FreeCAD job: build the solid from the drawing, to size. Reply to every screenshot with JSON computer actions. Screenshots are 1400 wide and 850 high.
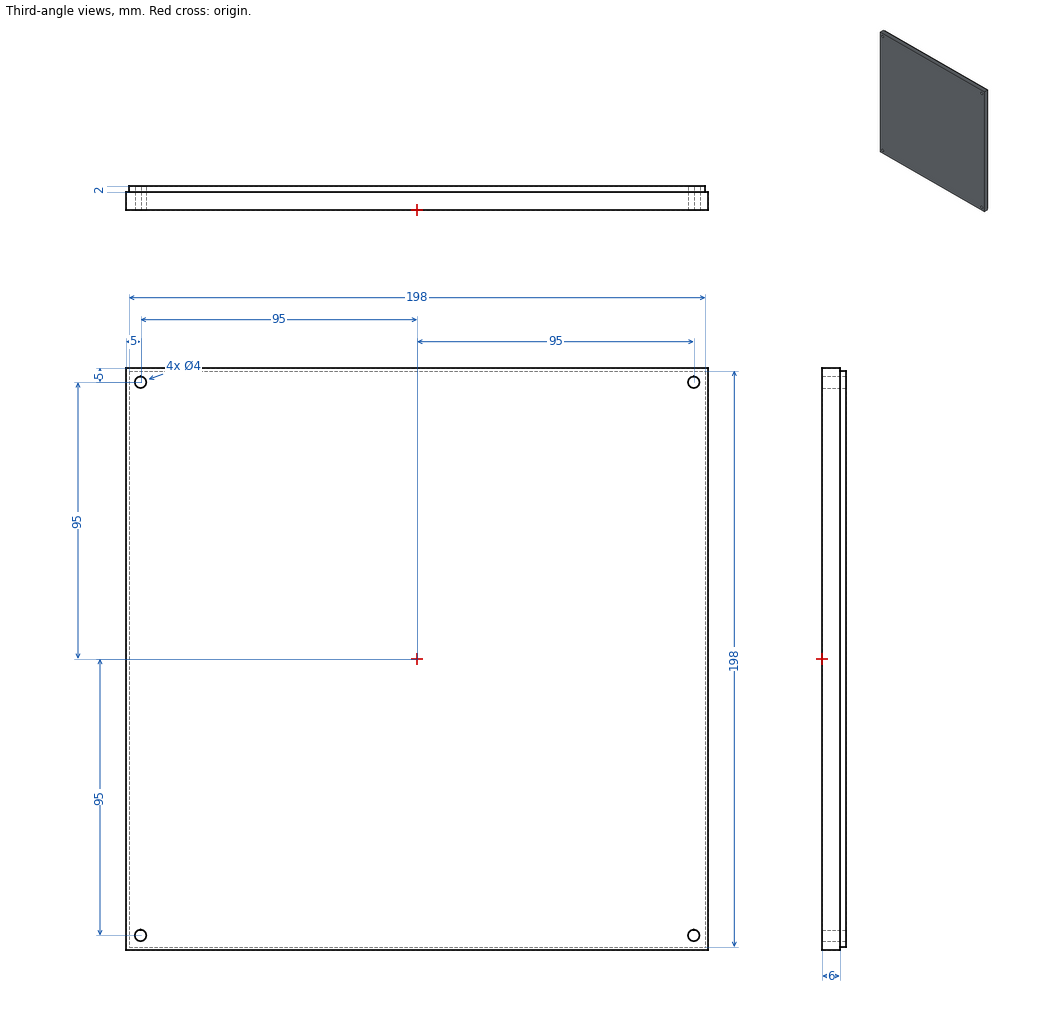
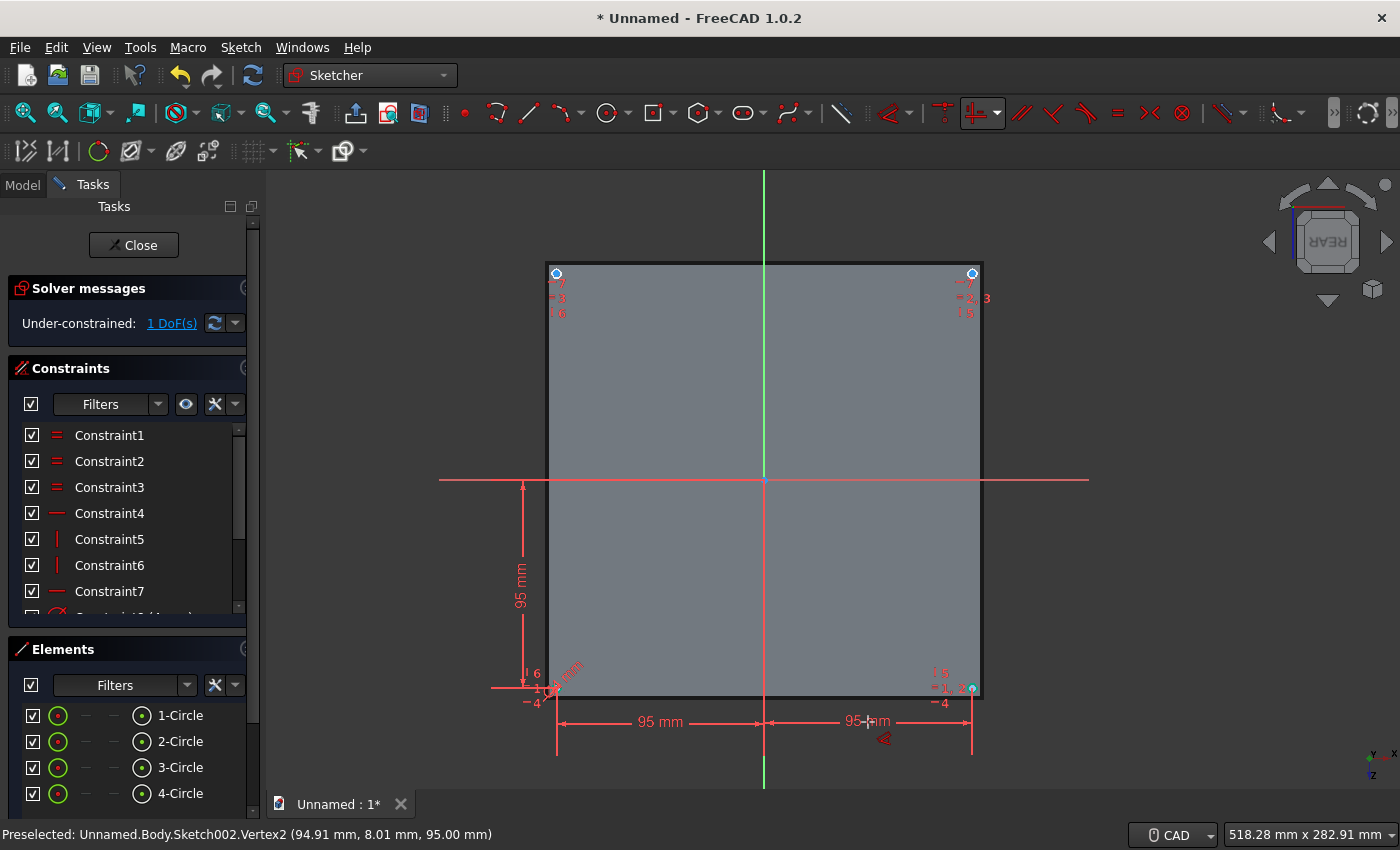
{"action": "left_click", "coordinate": [972, 274]}
{"action": "left_click", "coordinate": [1006, 377]}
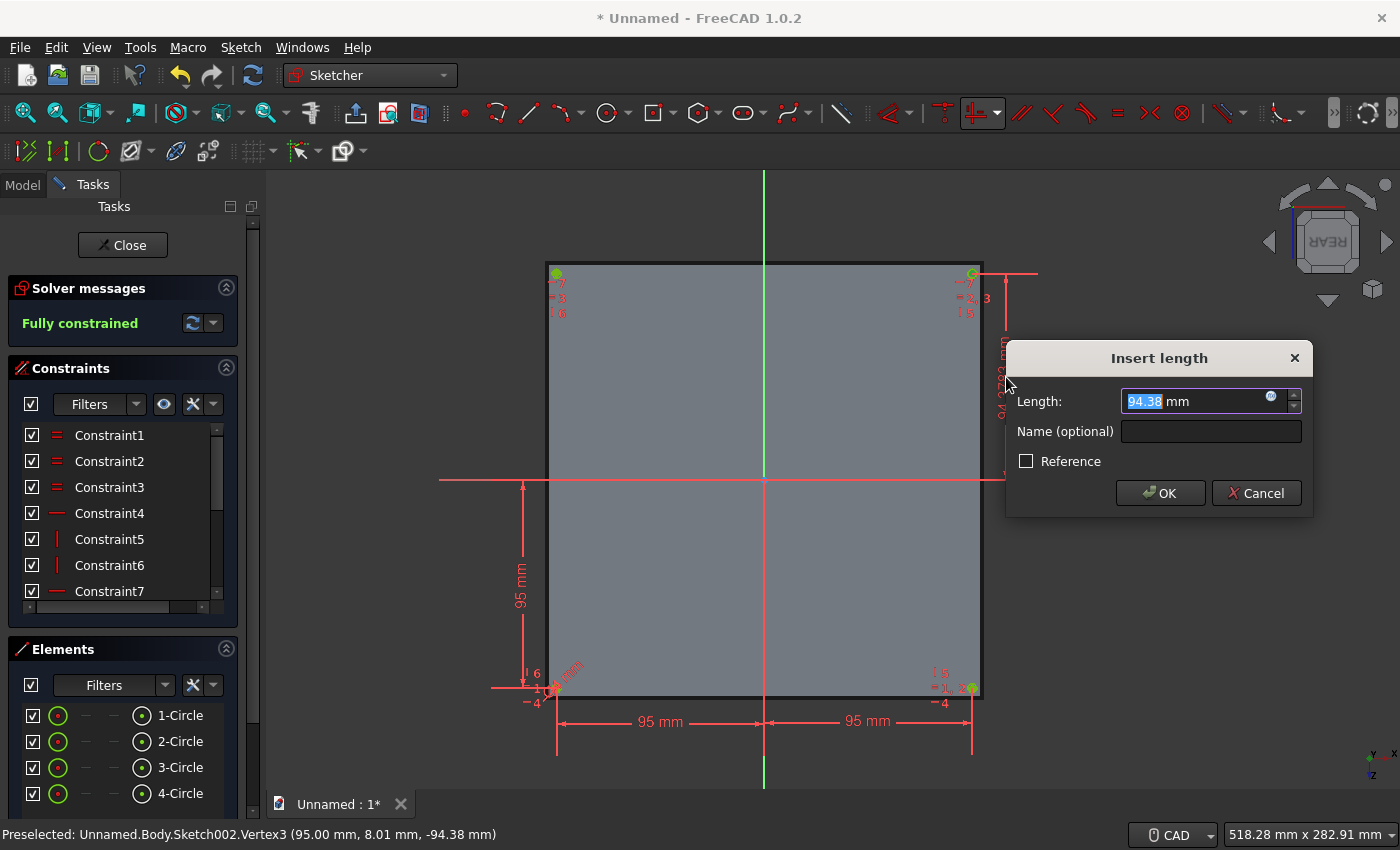
{"action": "type", "text": "95"}
{"action": "key", "text": "Return"}
{"action": "key", "text": "Escape"}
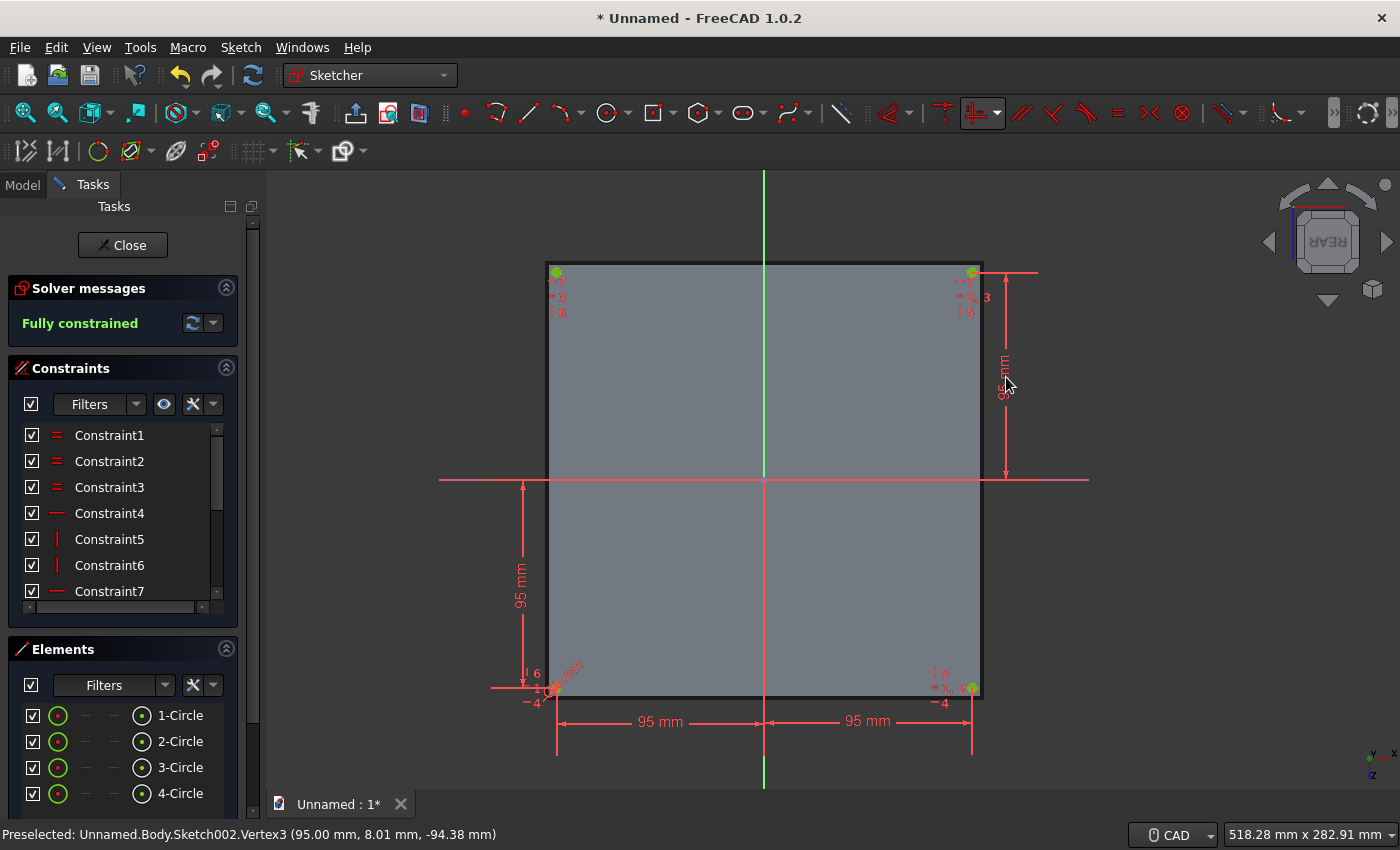
{"action": "left_click", "coordinate": [123, 245]}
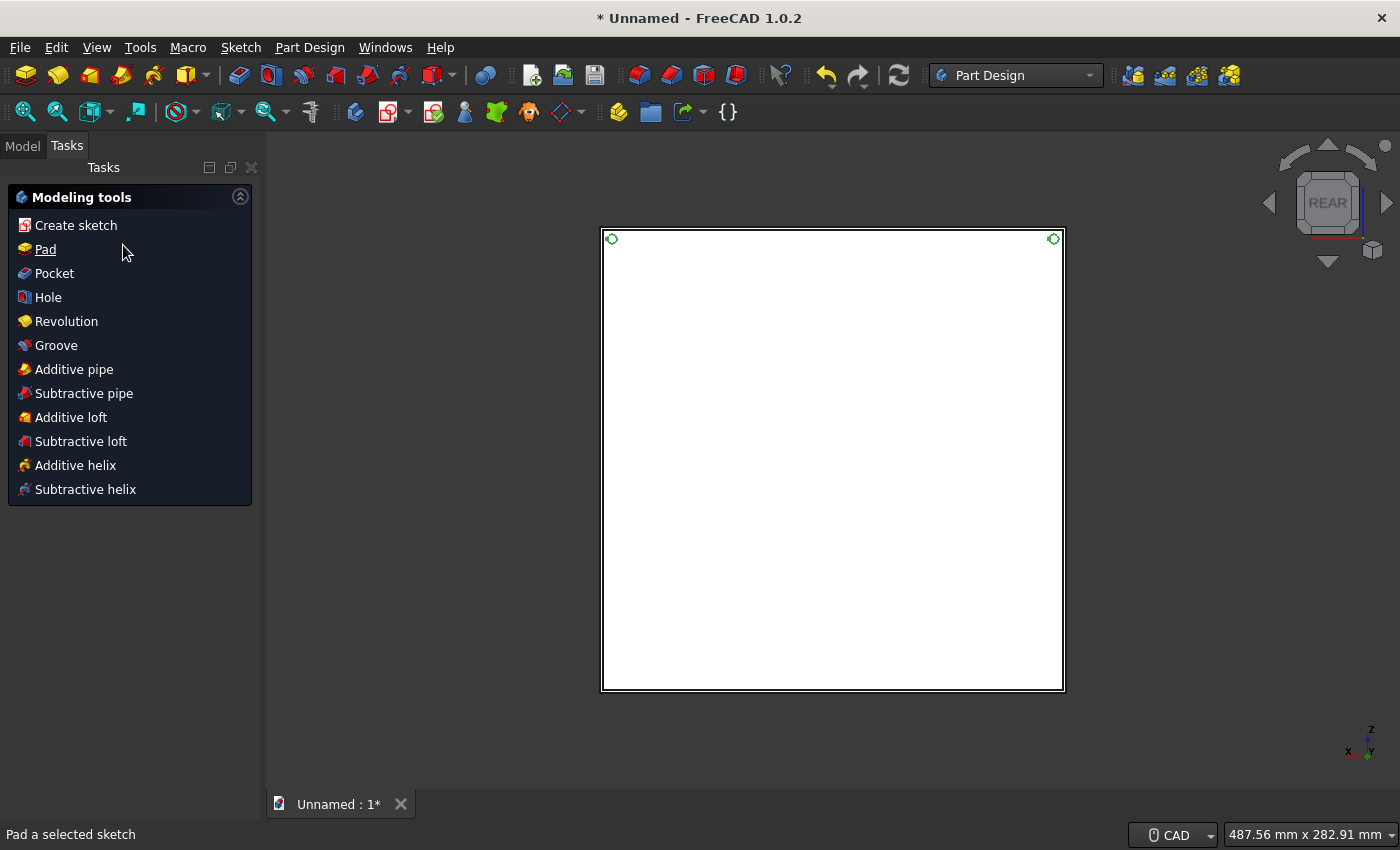
{"action": "left_click", "coordinate": [240, 76]}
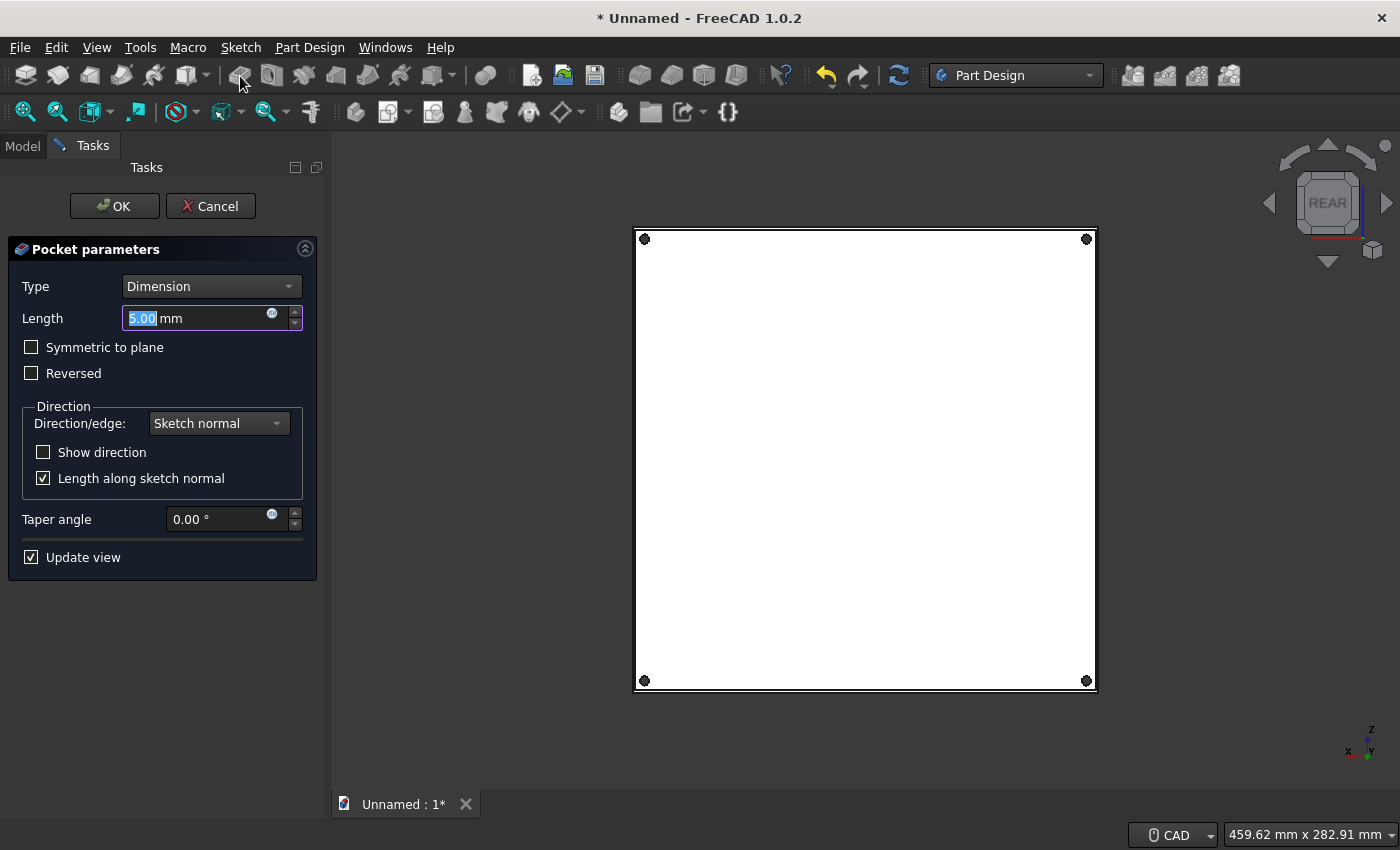
{"action": "left_click", "coordinate": [212, 286]}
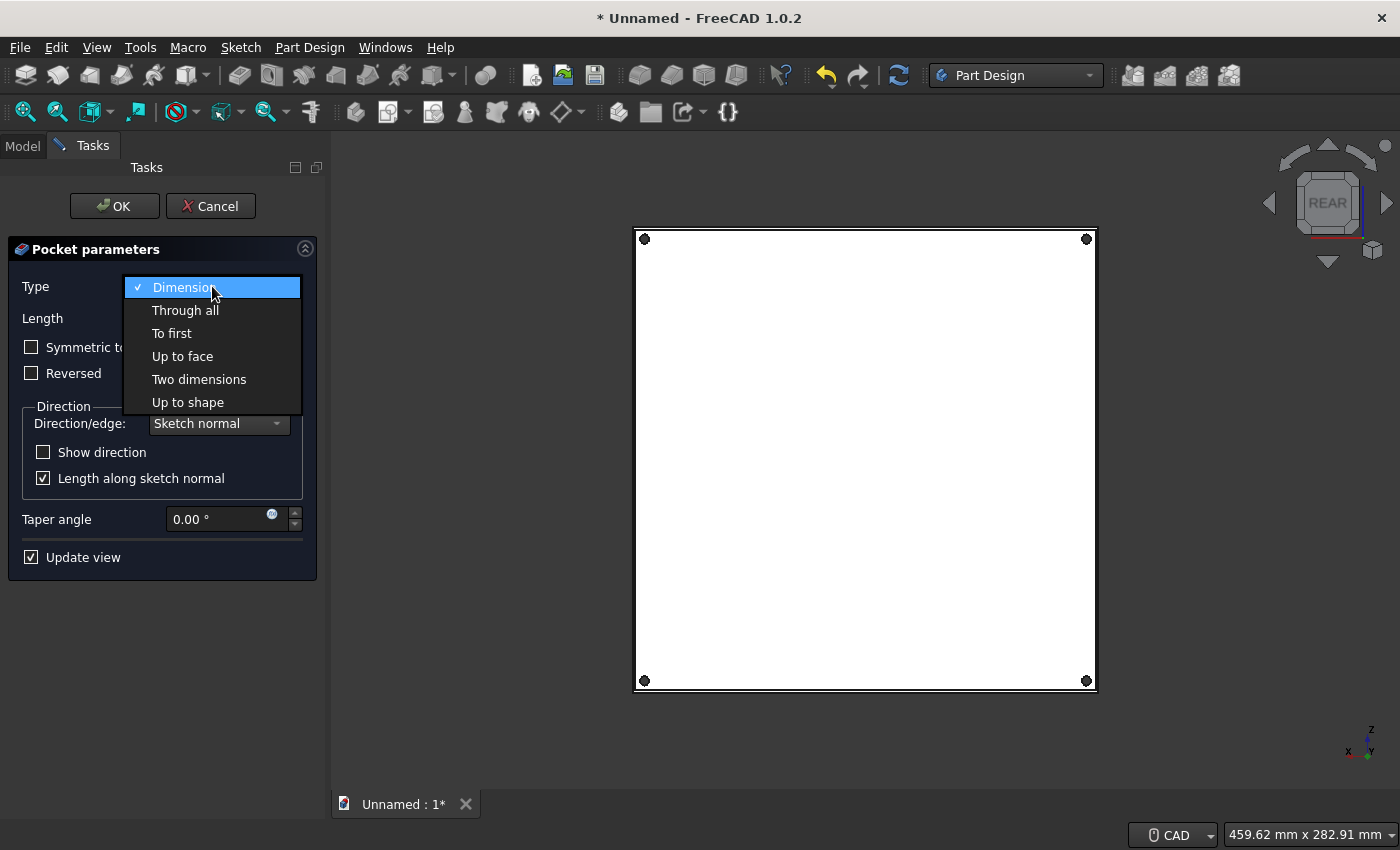
{"action": "left_click", "coordinate": [212, 310]}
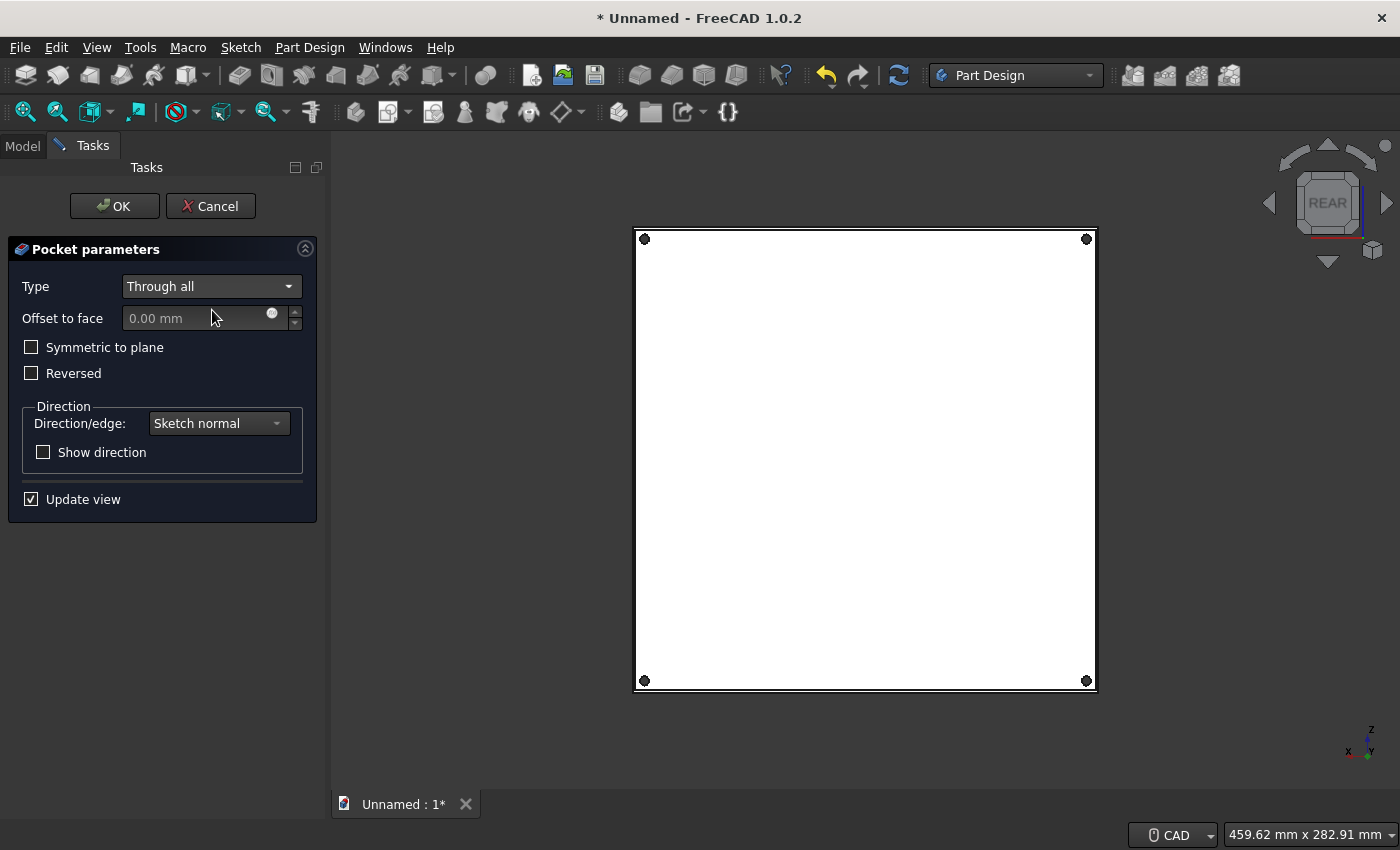
{"action": "left_click", "coordinate": [115, 206]}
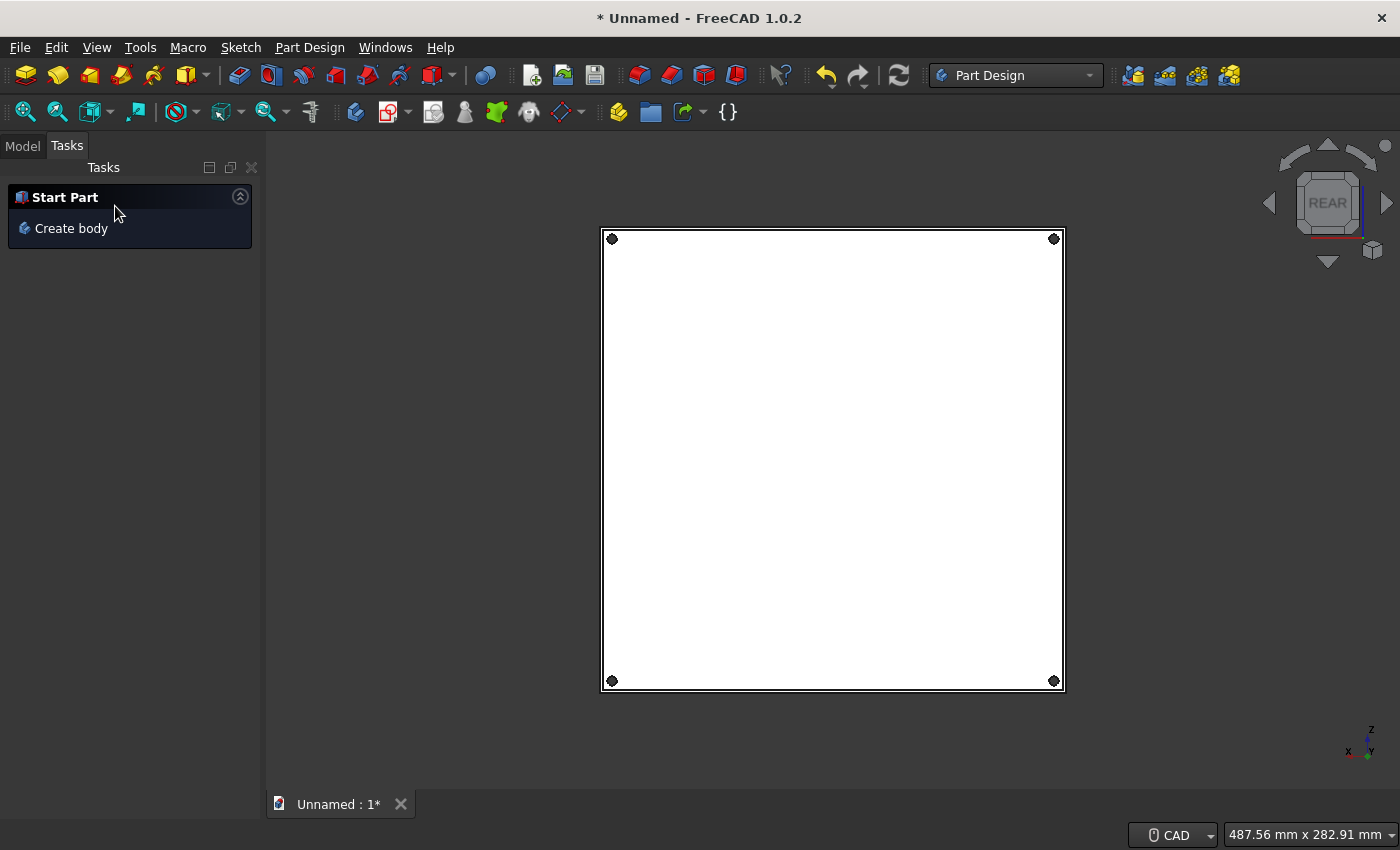
{"action": "key", "text": "0"}